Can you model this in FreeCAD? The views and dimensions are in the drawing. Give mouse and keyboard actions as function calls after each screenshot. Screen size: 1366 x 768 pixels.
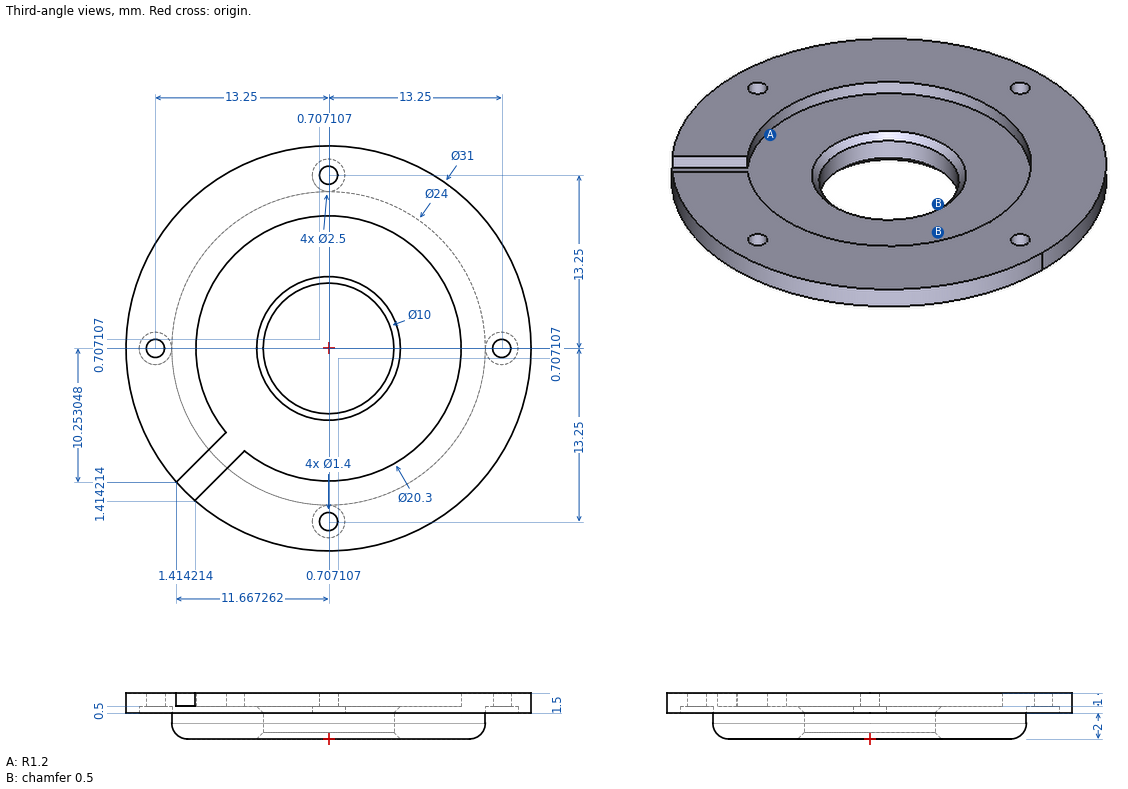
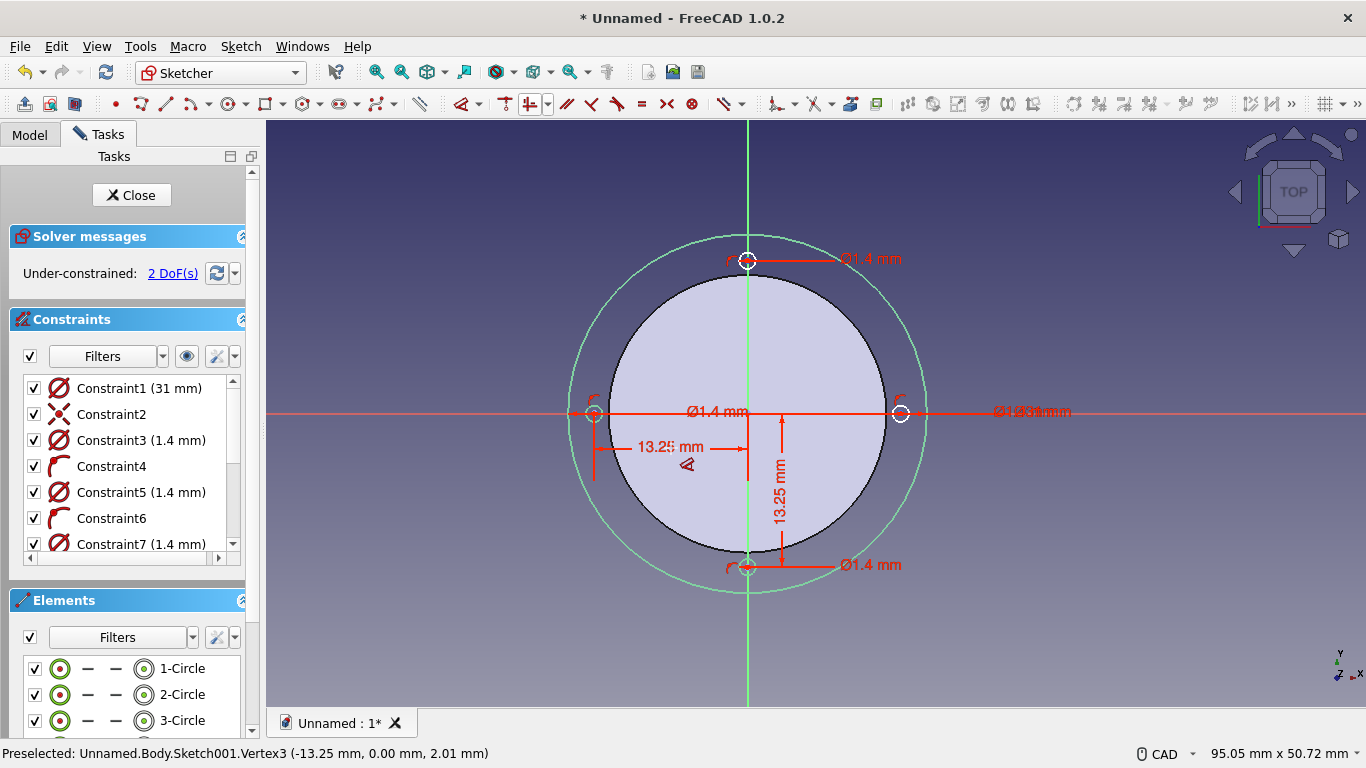
click(901, 414)
click(824, 448)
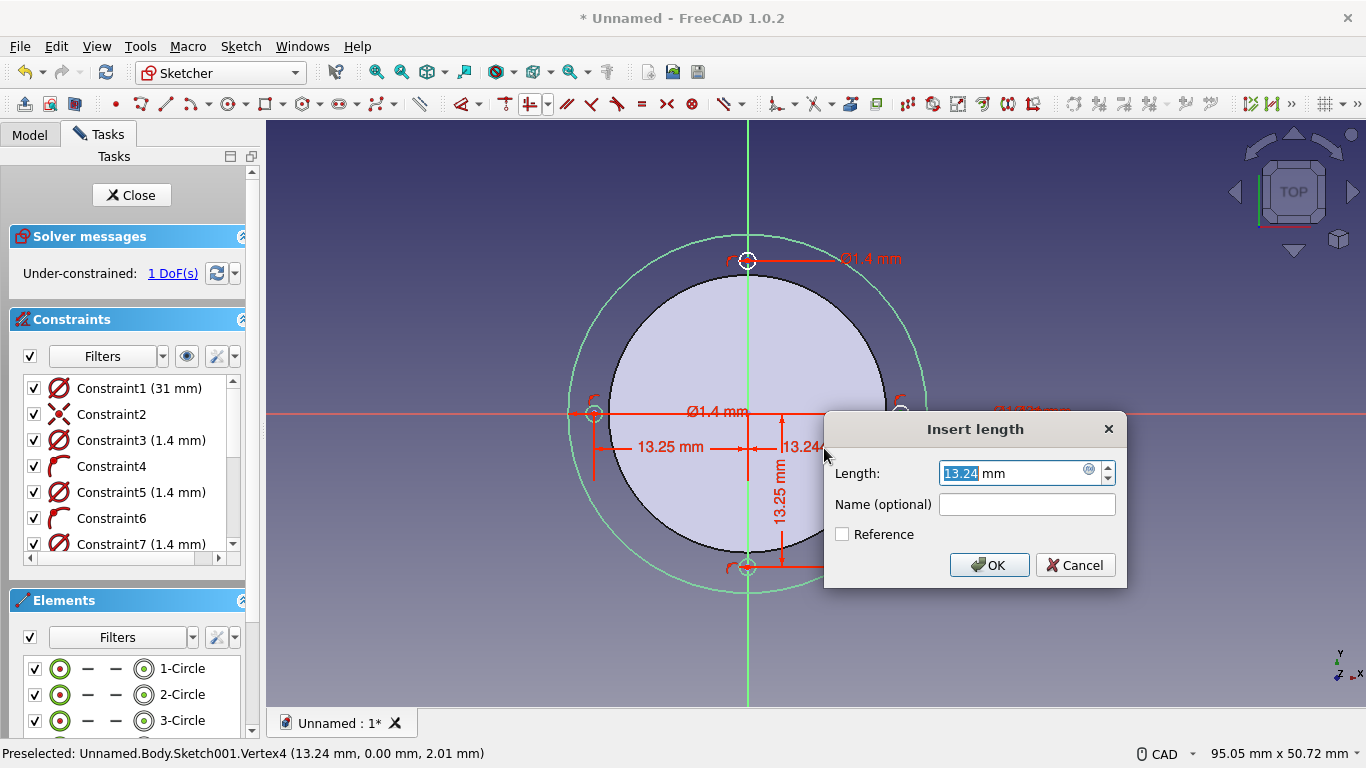
text(13.25)
key(Return)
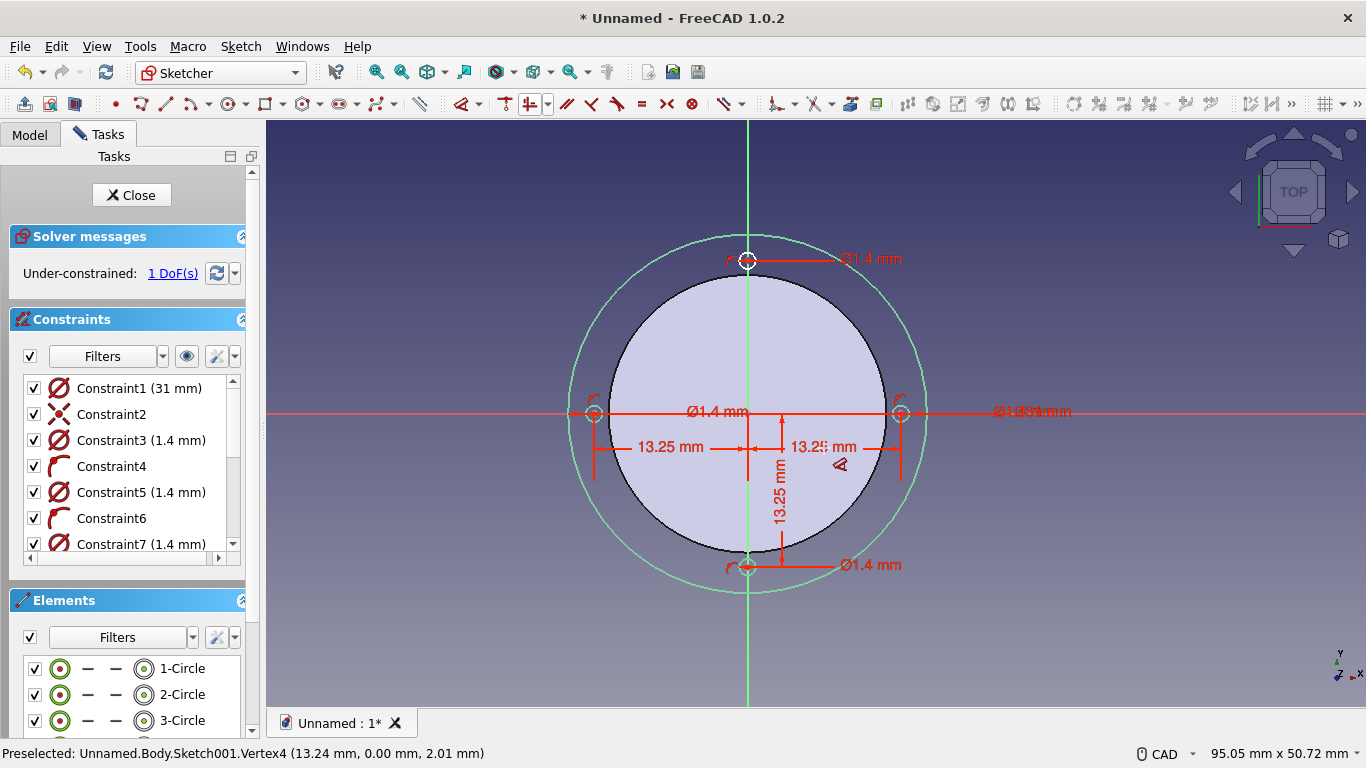
click(748, 261)
click(782, 337)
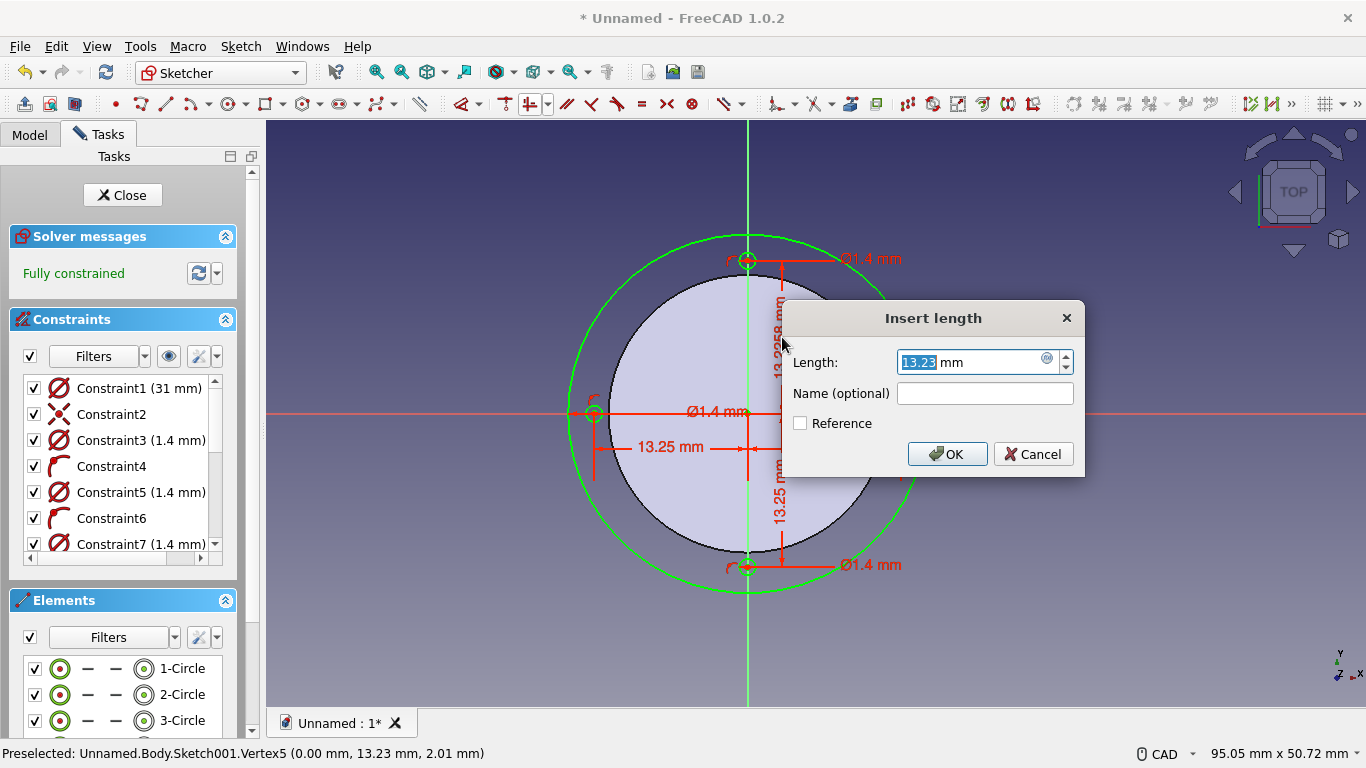
text(13.25)
key(Return)
key(Escape)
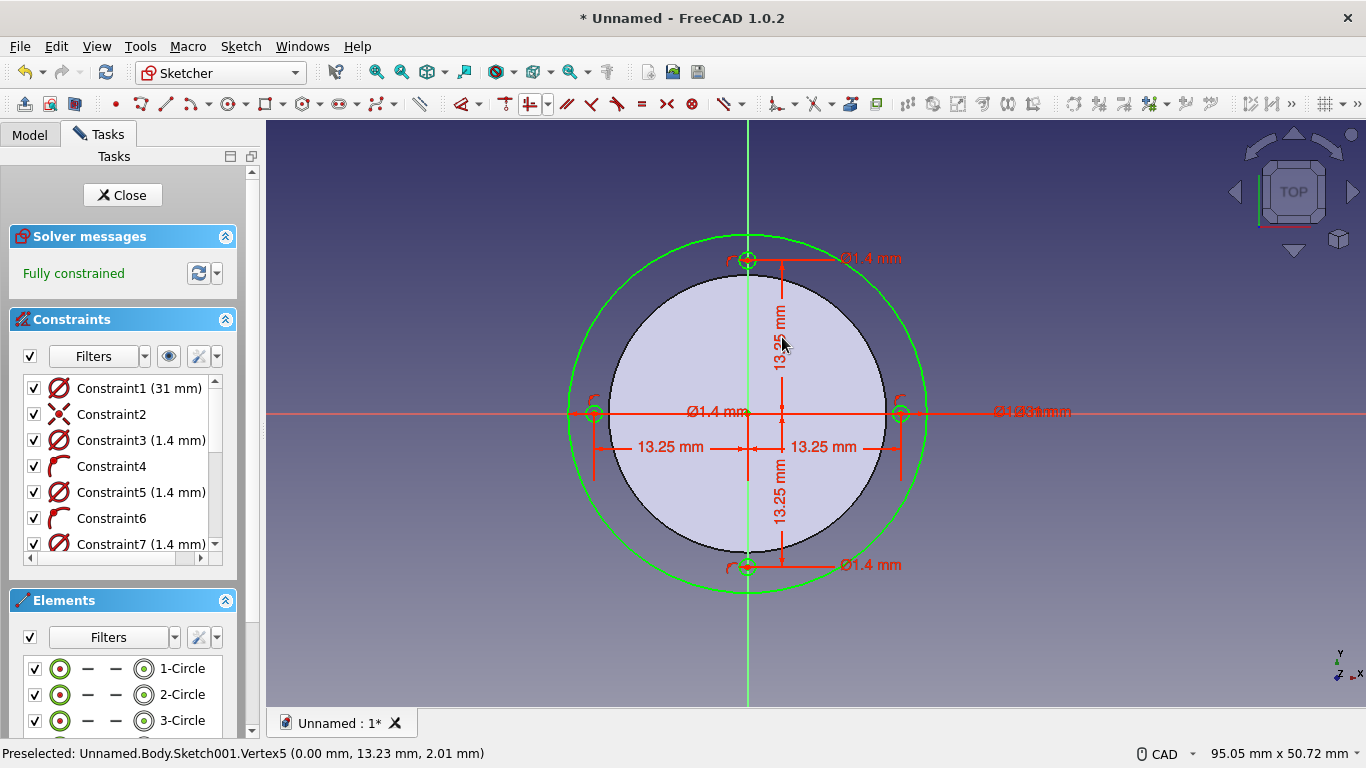
click(123, 195)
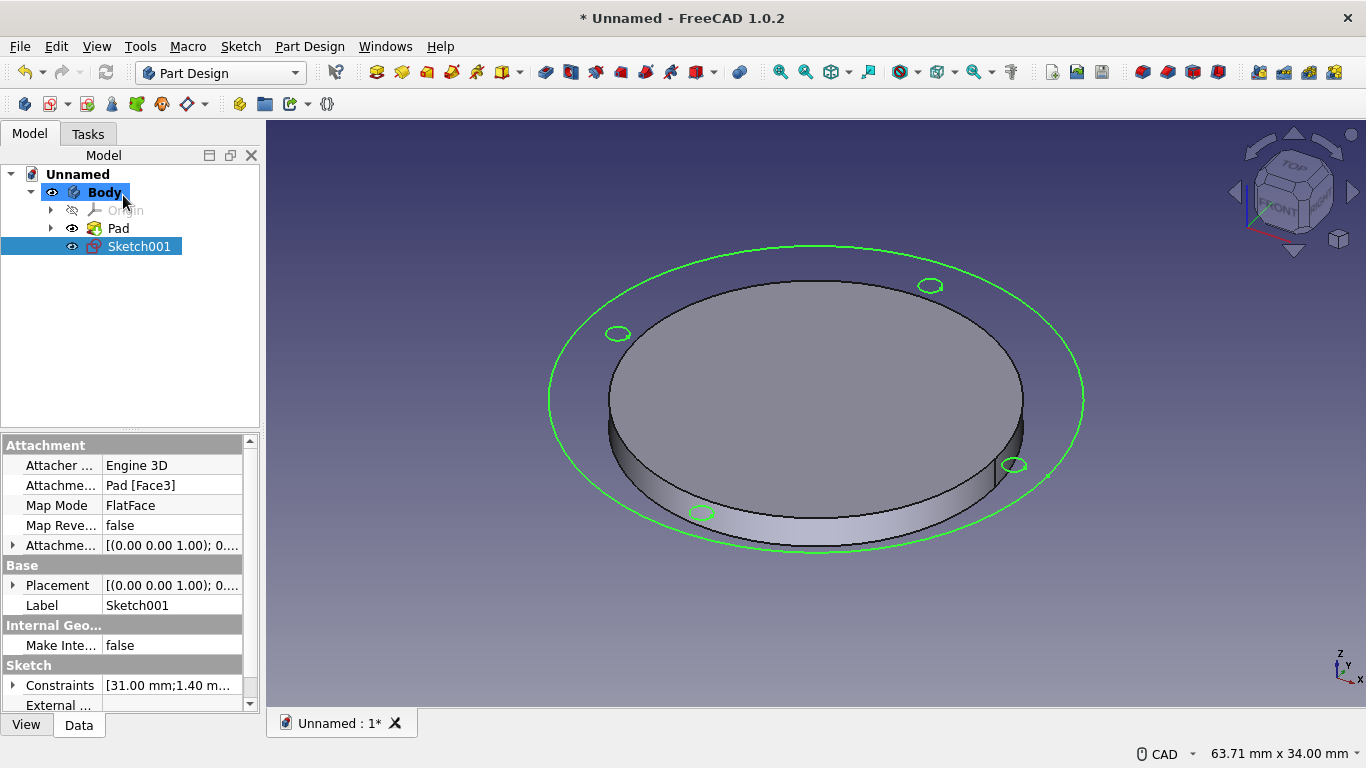
click(377, 72)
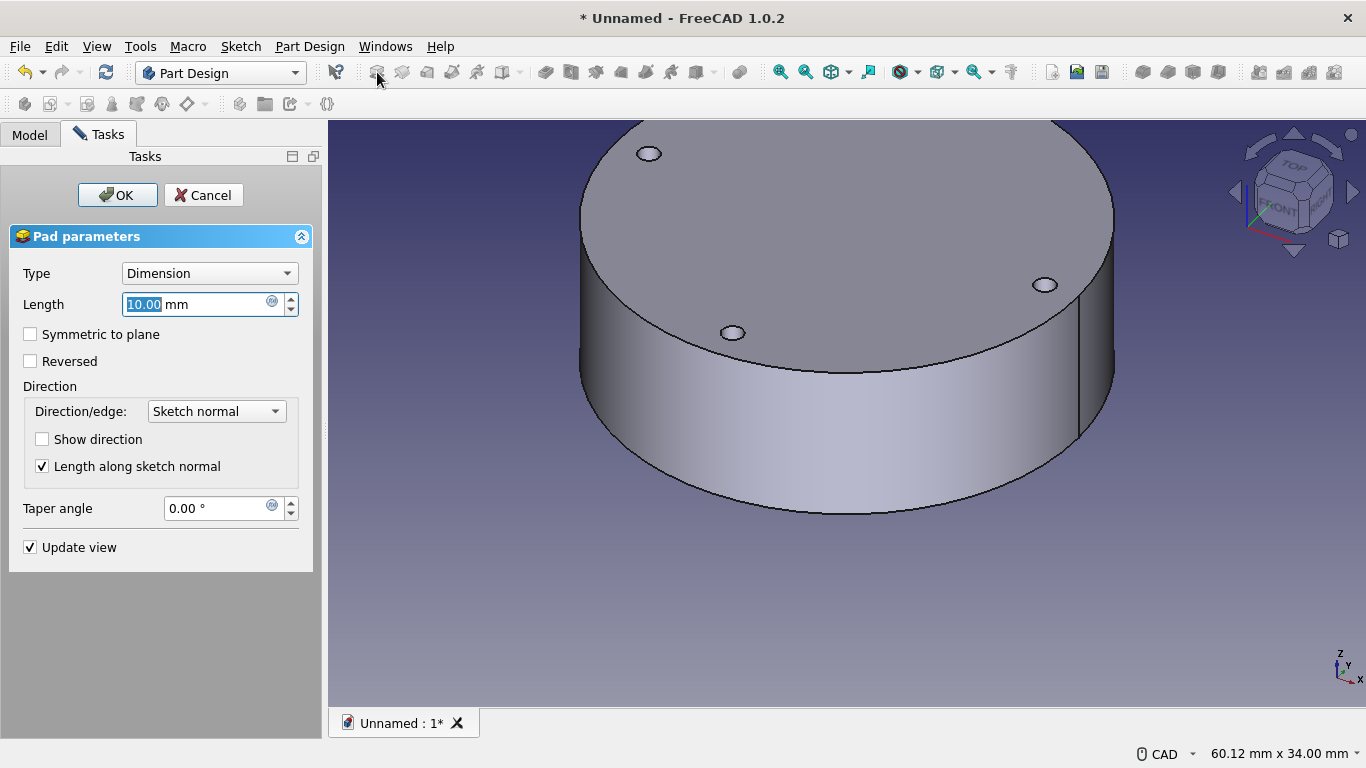
text(1.5)
key(Tab)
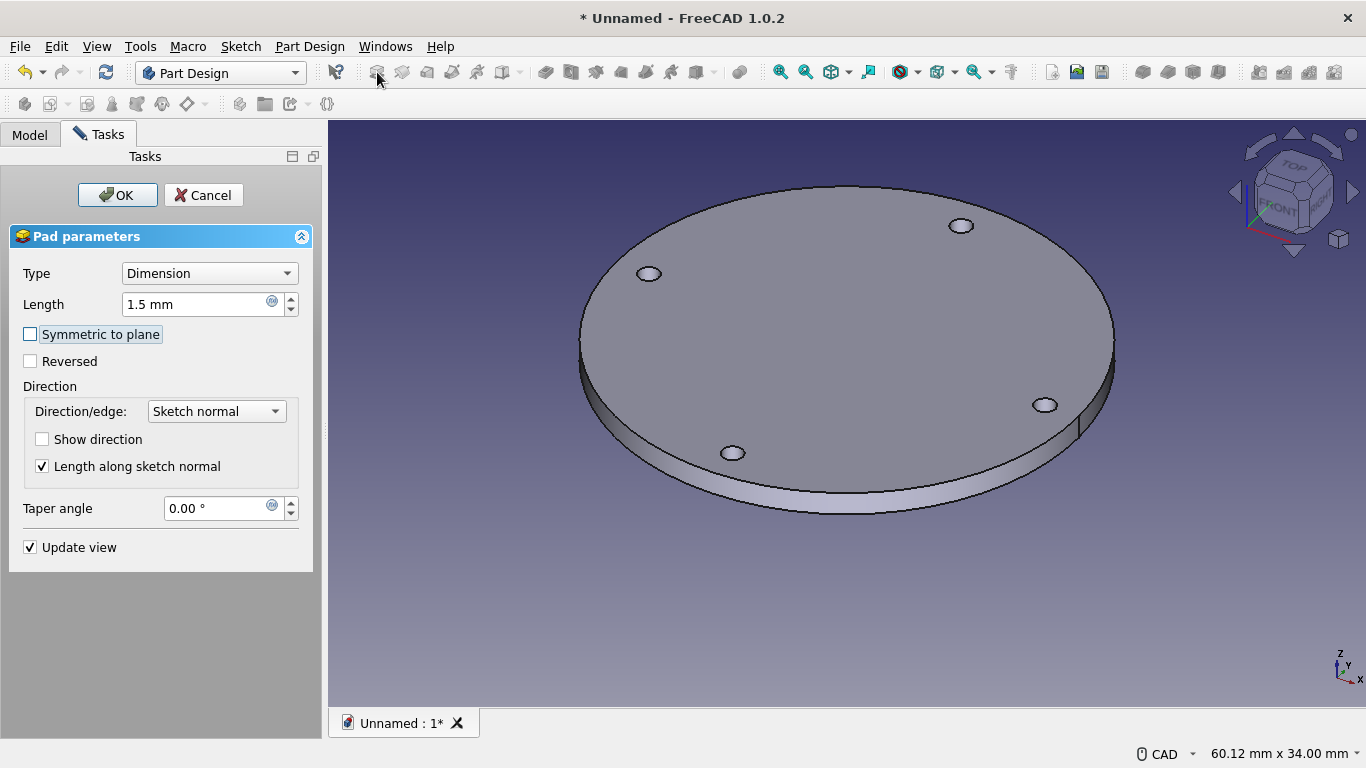
click(118, 195)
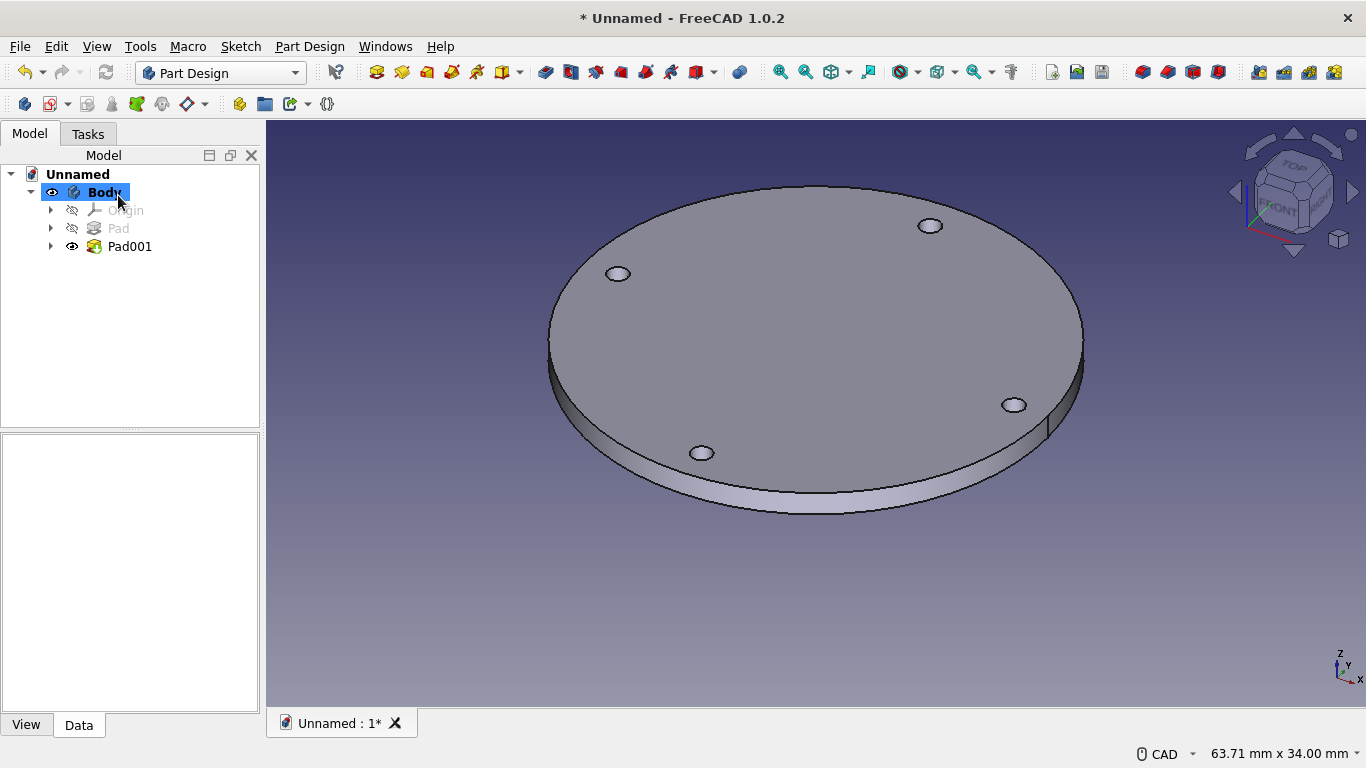
click(816, 339)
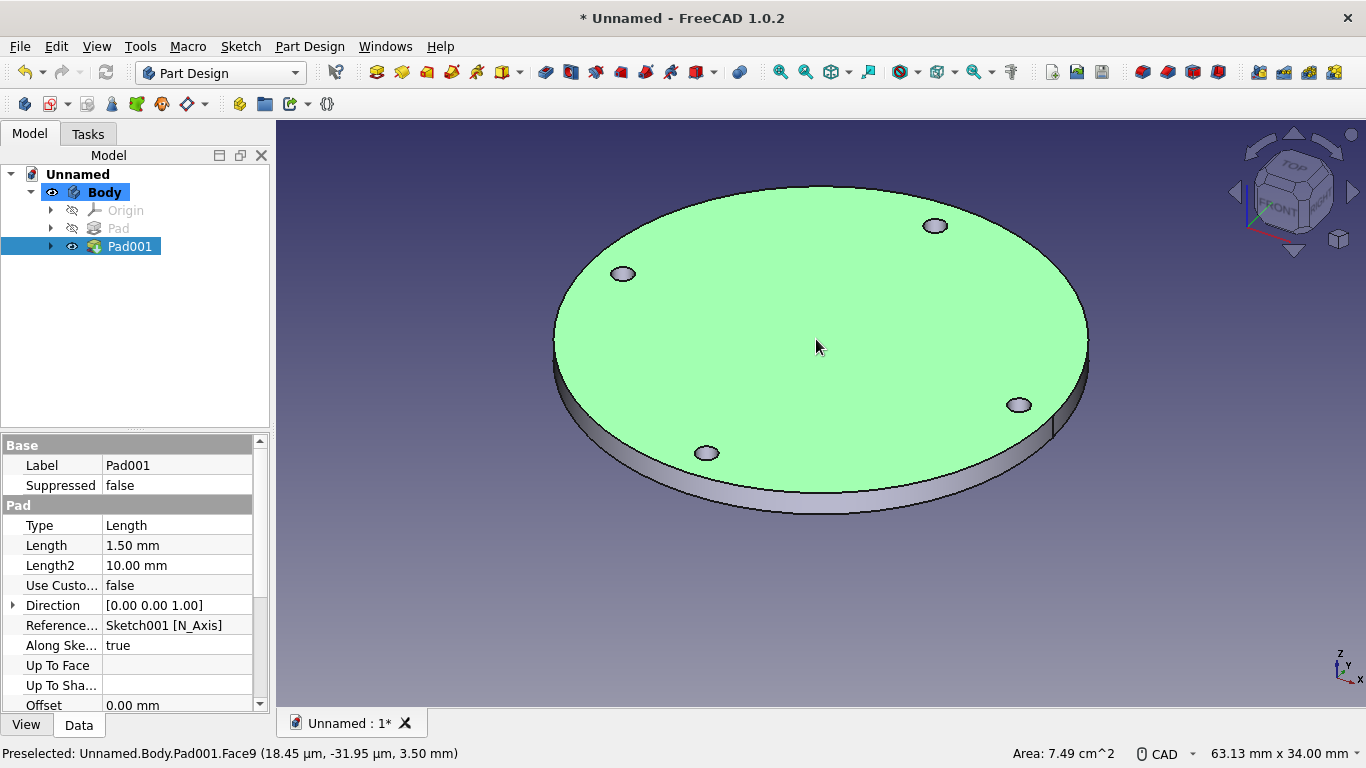
click(50, 104)